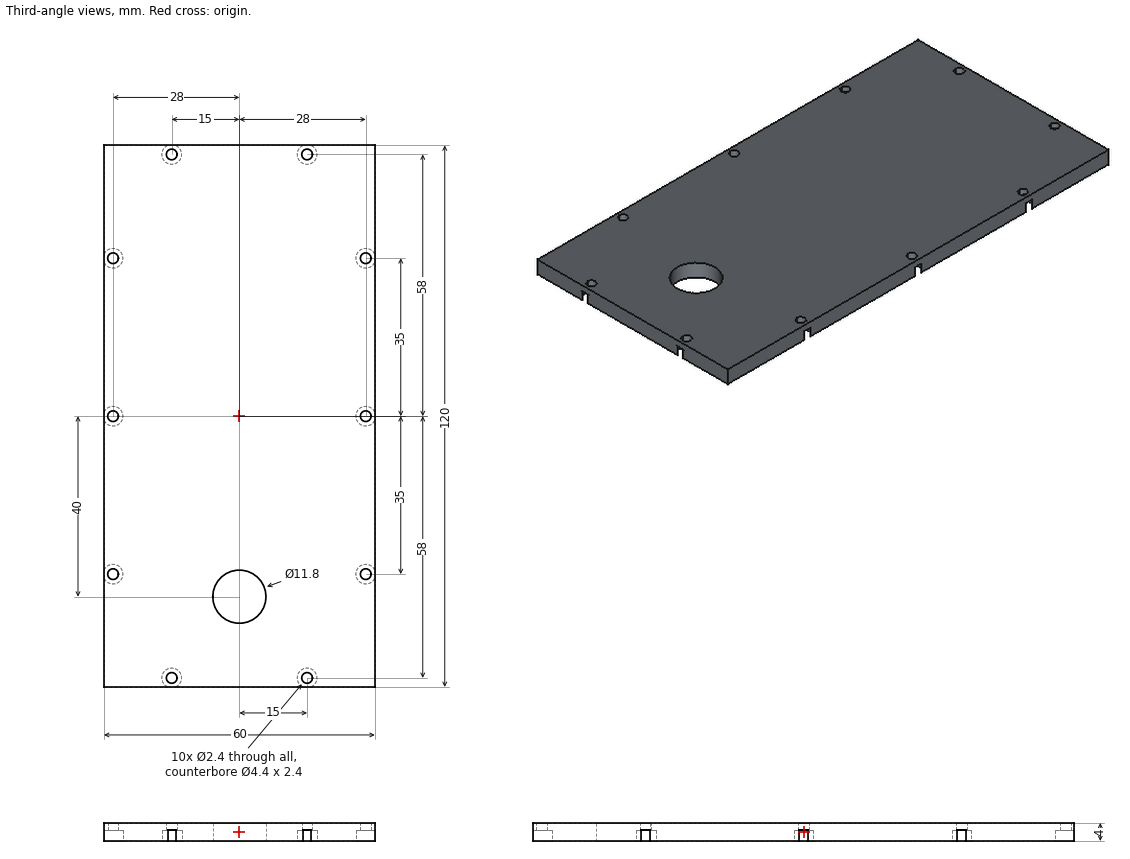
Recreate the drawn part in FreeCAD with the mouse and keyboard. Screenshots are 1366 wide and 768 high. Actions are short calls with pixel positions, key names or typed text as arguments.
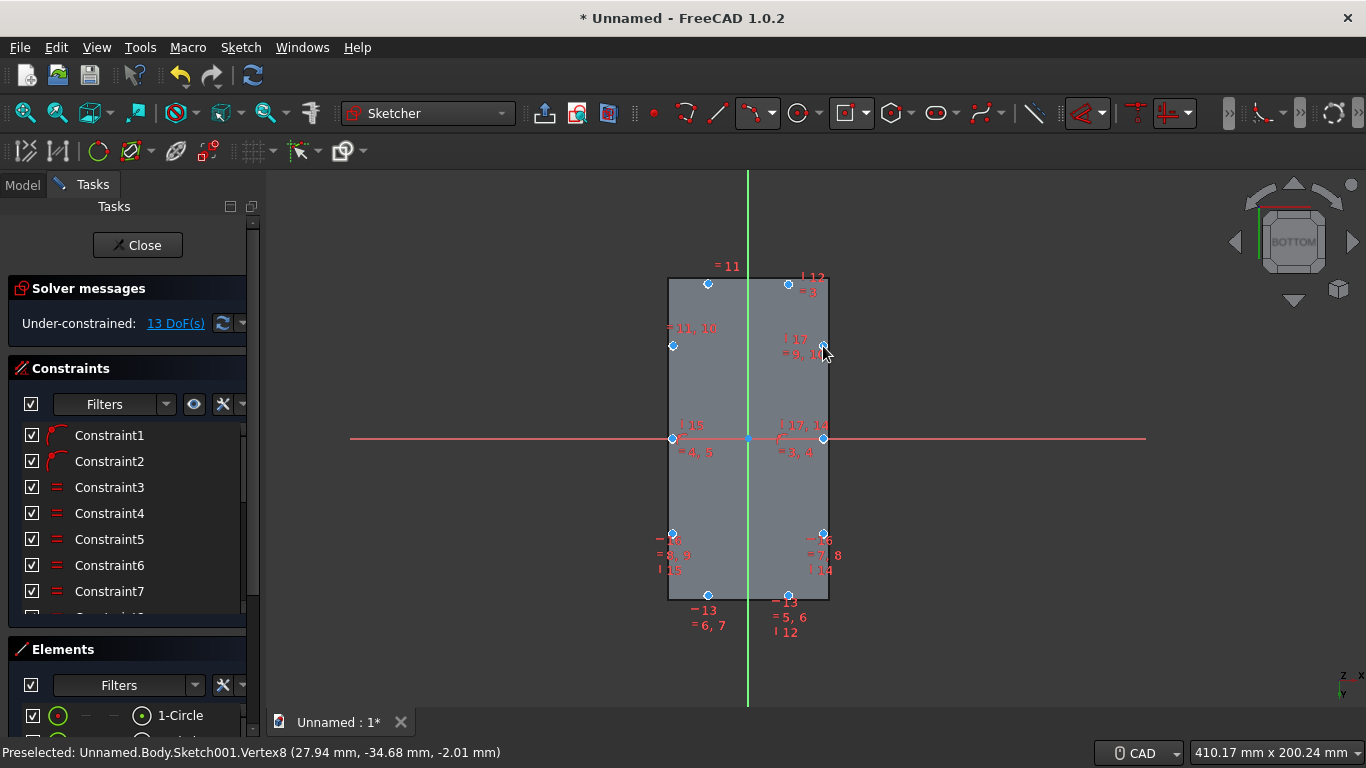
click(673, 439)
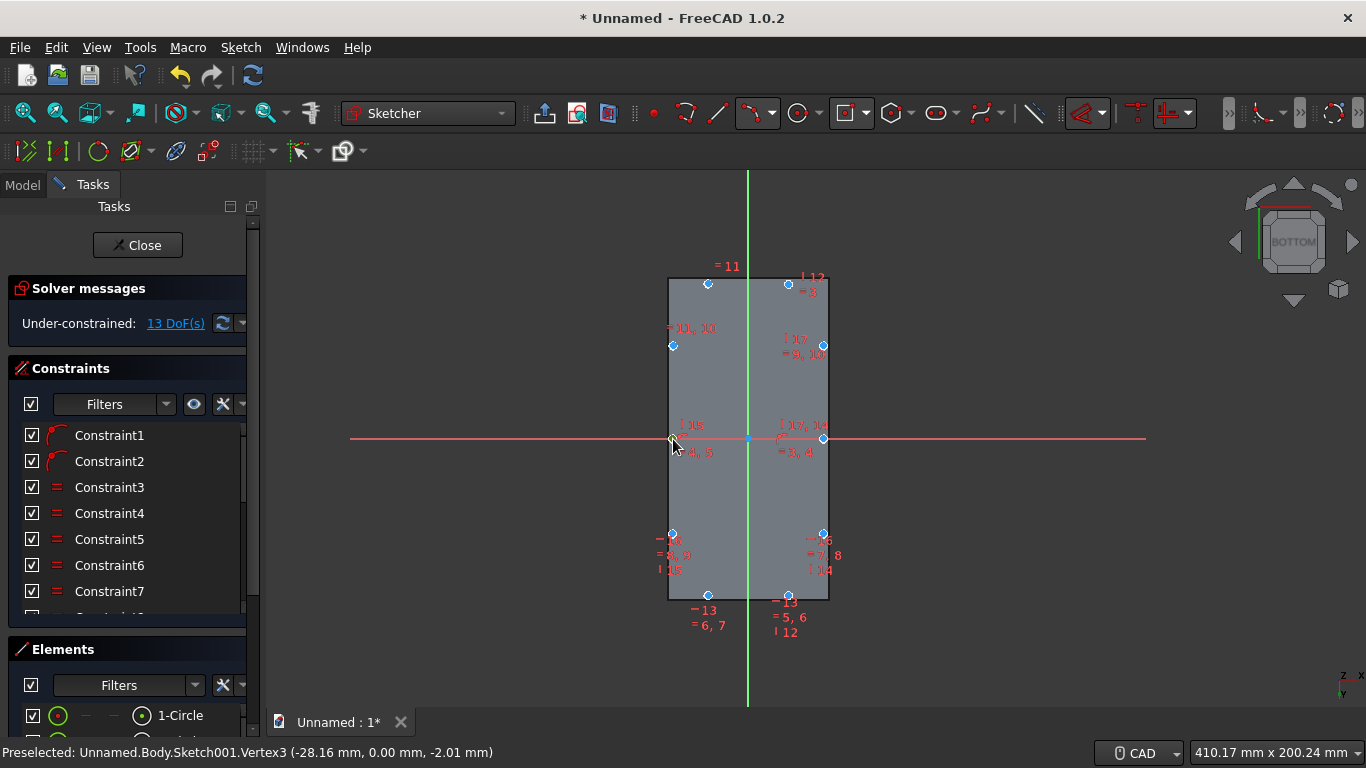
click(673, 346)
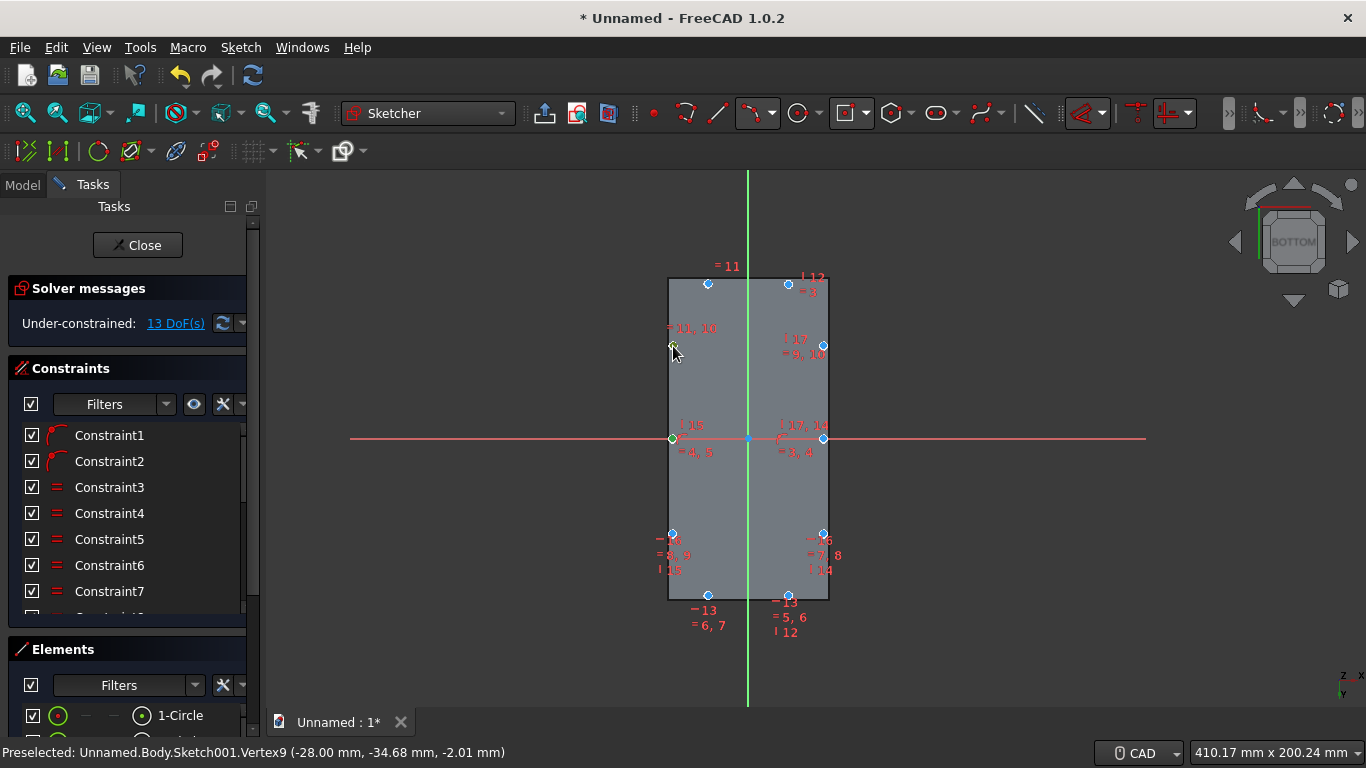
click(1190, 114)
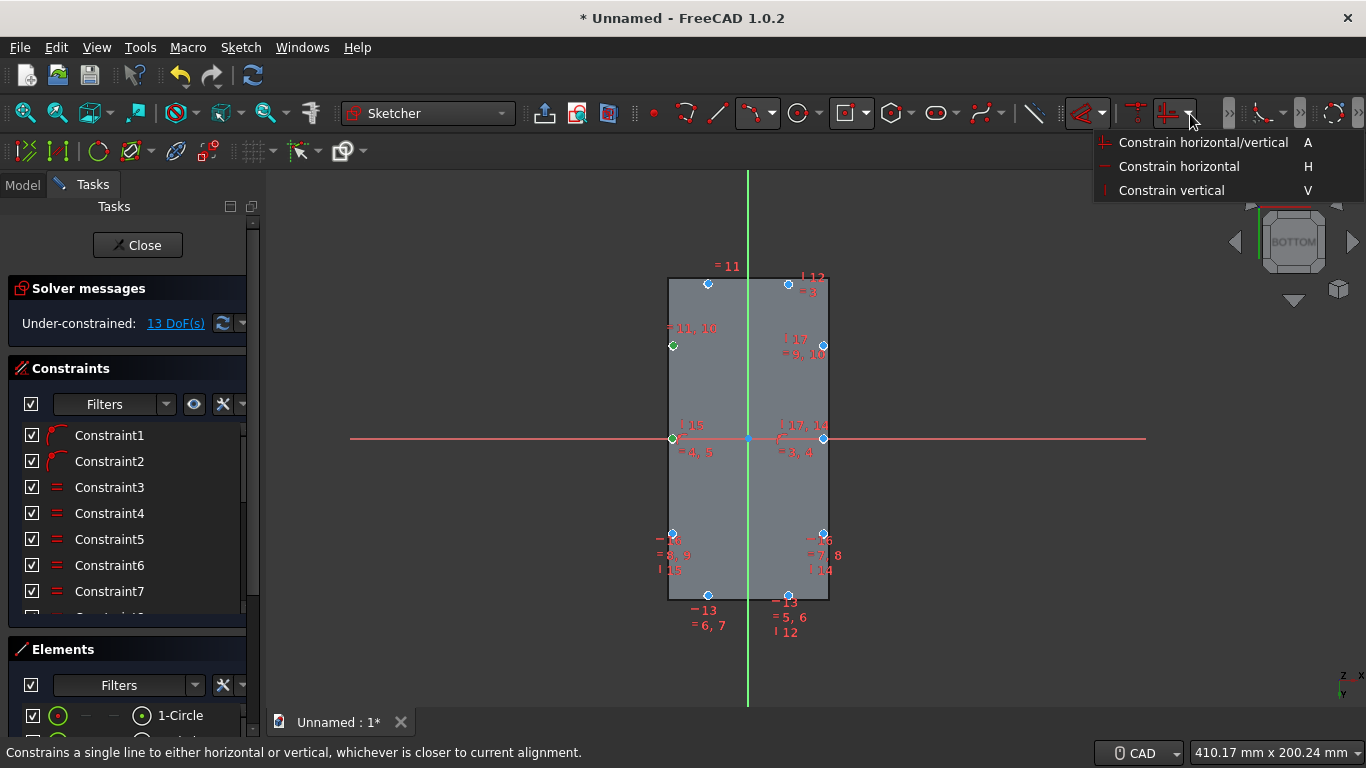
click(1229, 190)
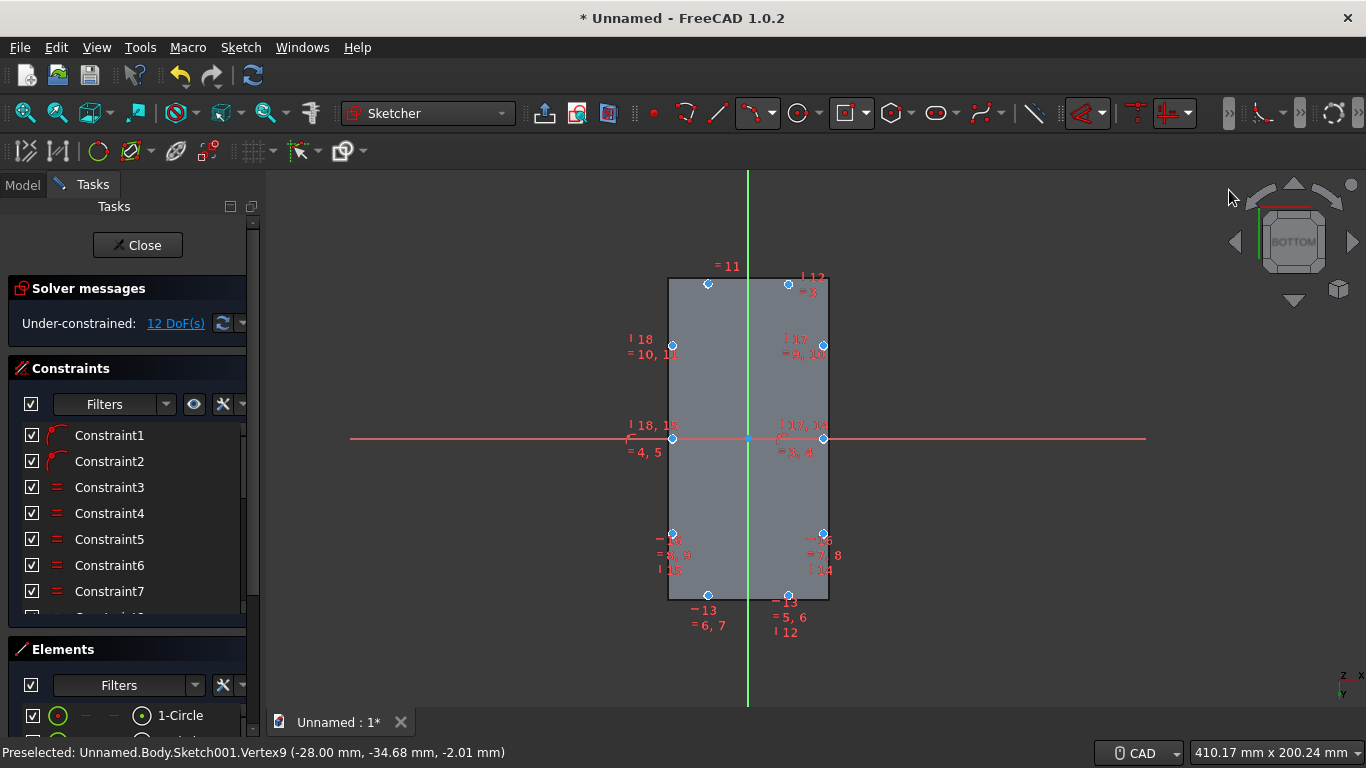
click(826, 348)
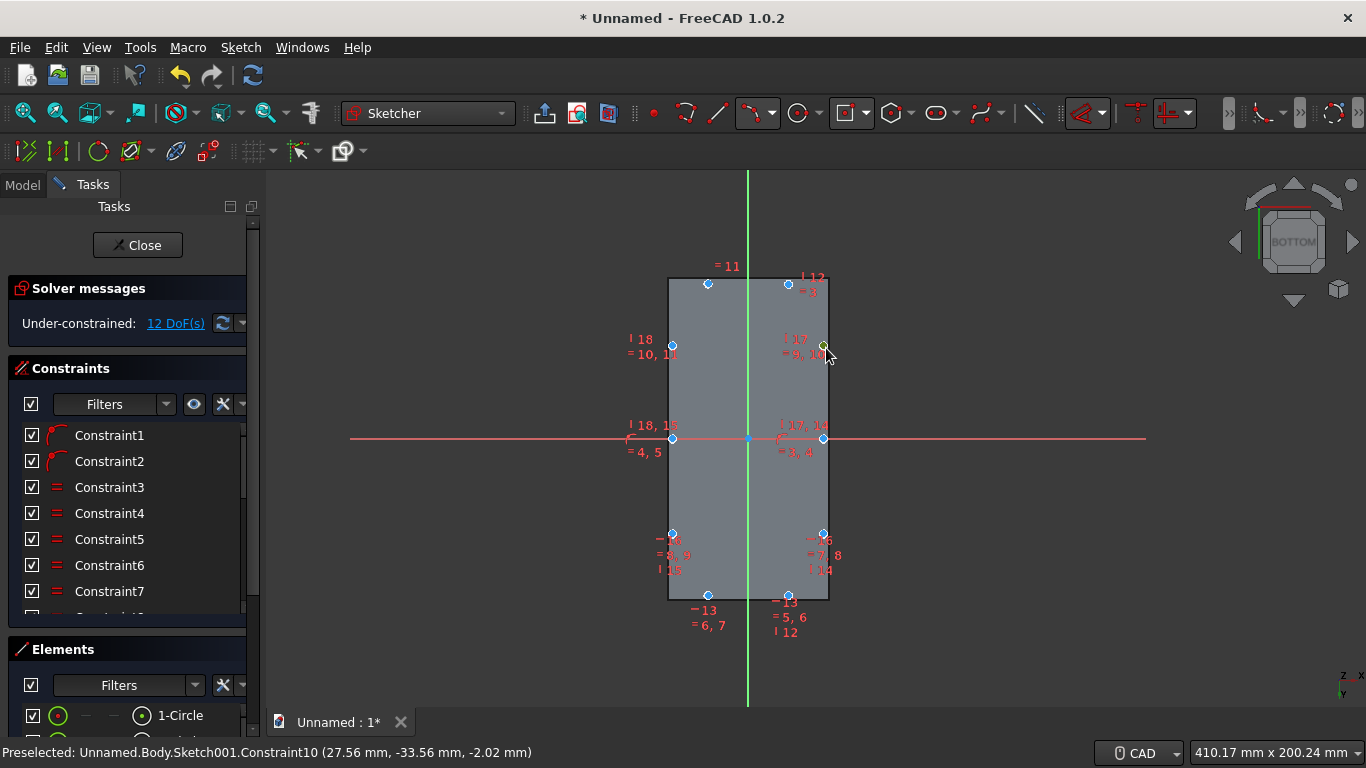
scroll(673, 346, up, 4)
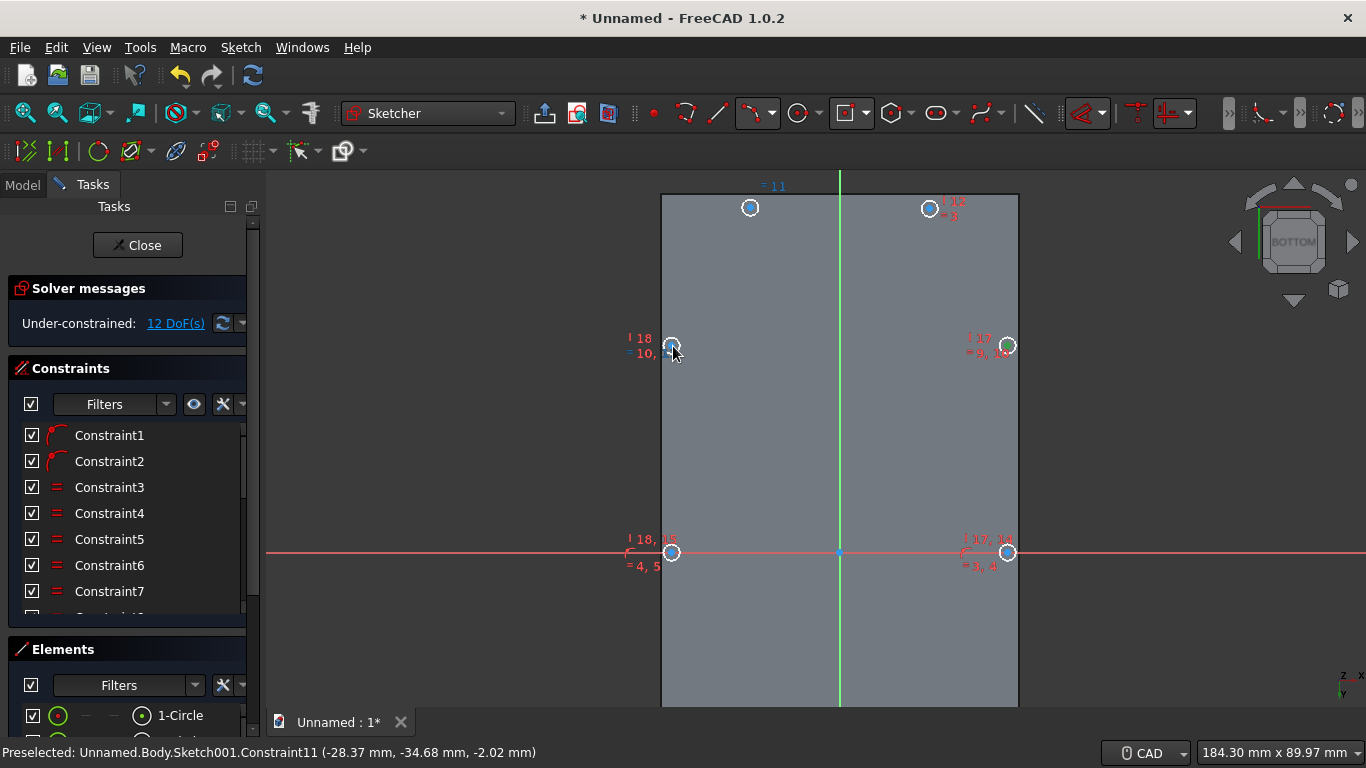
scroll(672, 346, up, 4)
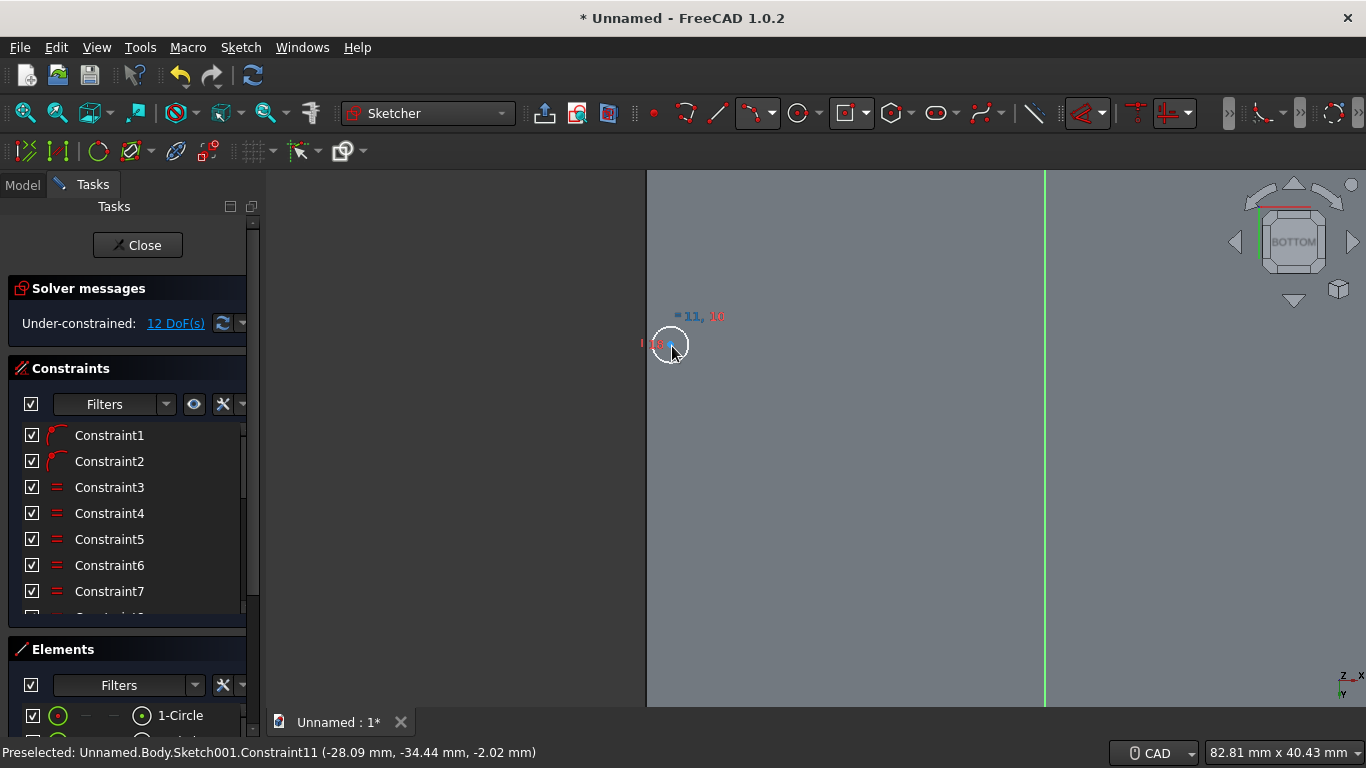
click(671, 345)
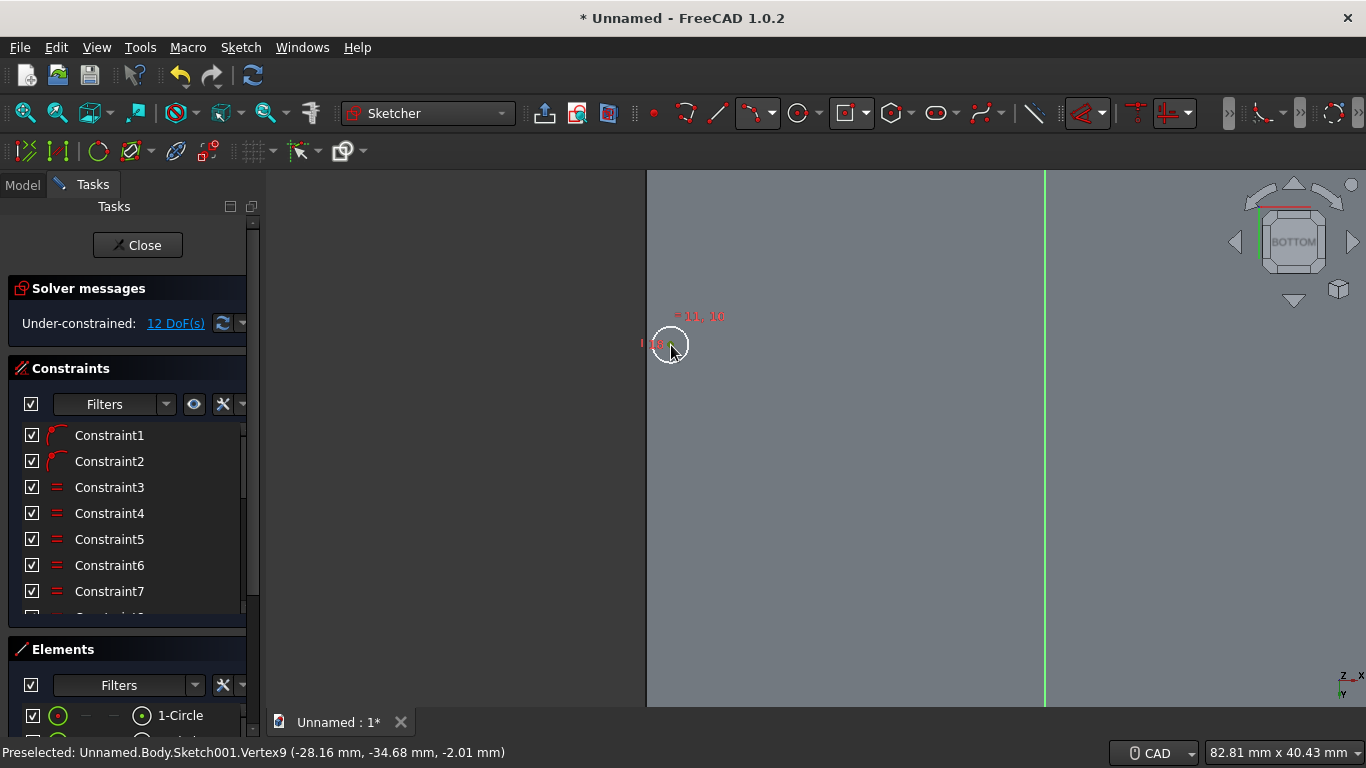
key(h)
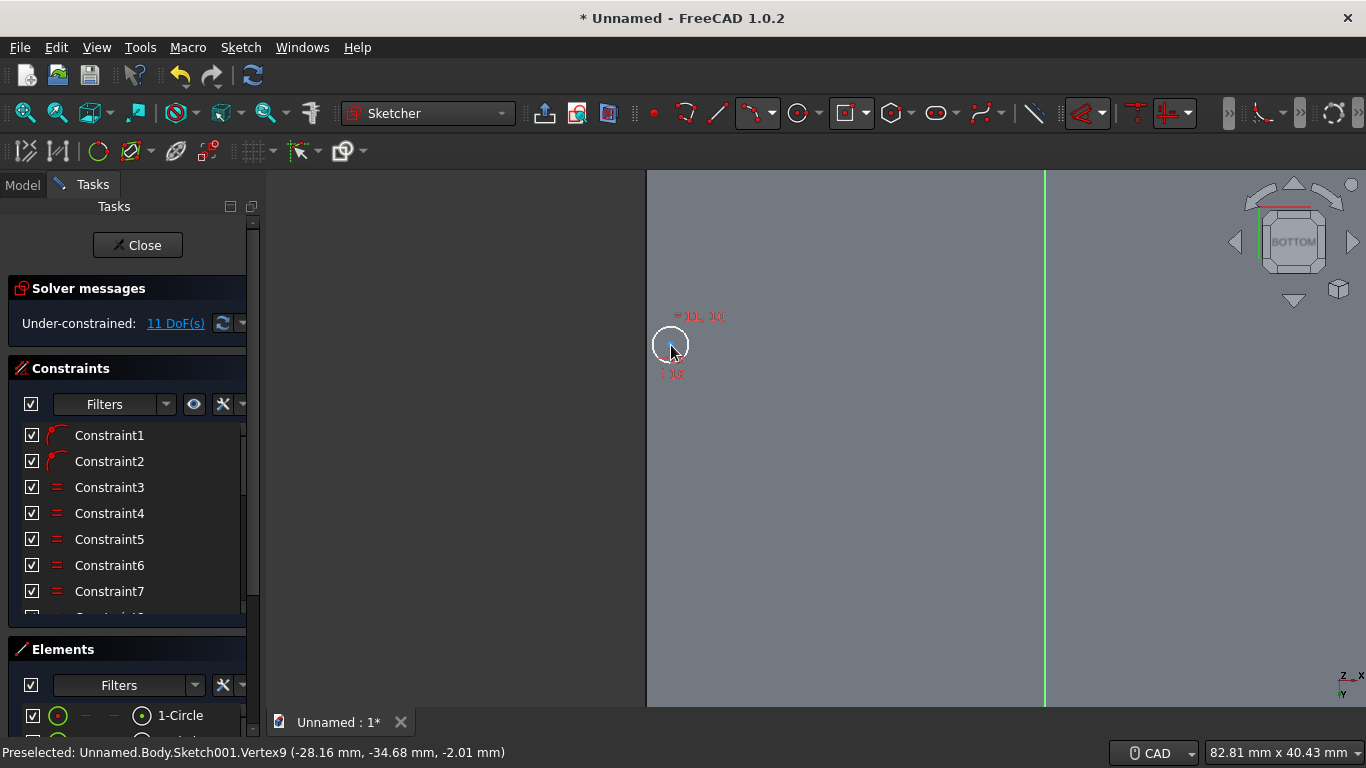
scroll(672, 346, down, 8)